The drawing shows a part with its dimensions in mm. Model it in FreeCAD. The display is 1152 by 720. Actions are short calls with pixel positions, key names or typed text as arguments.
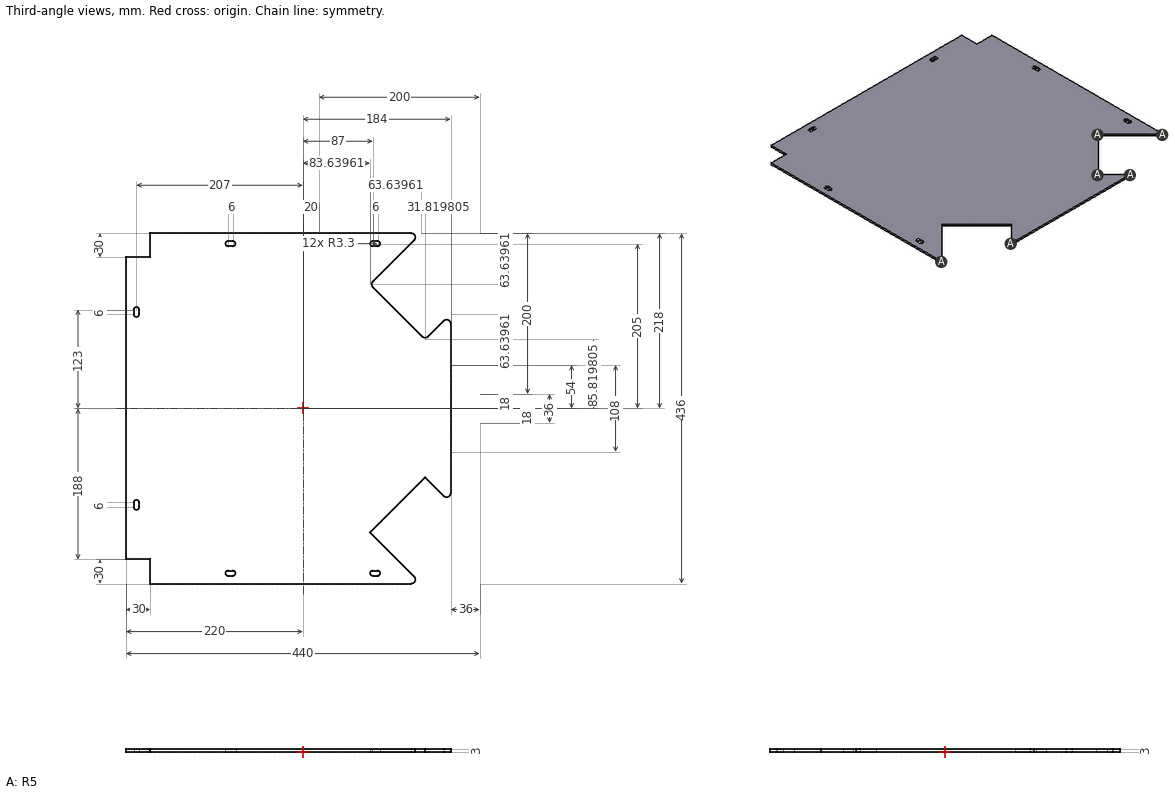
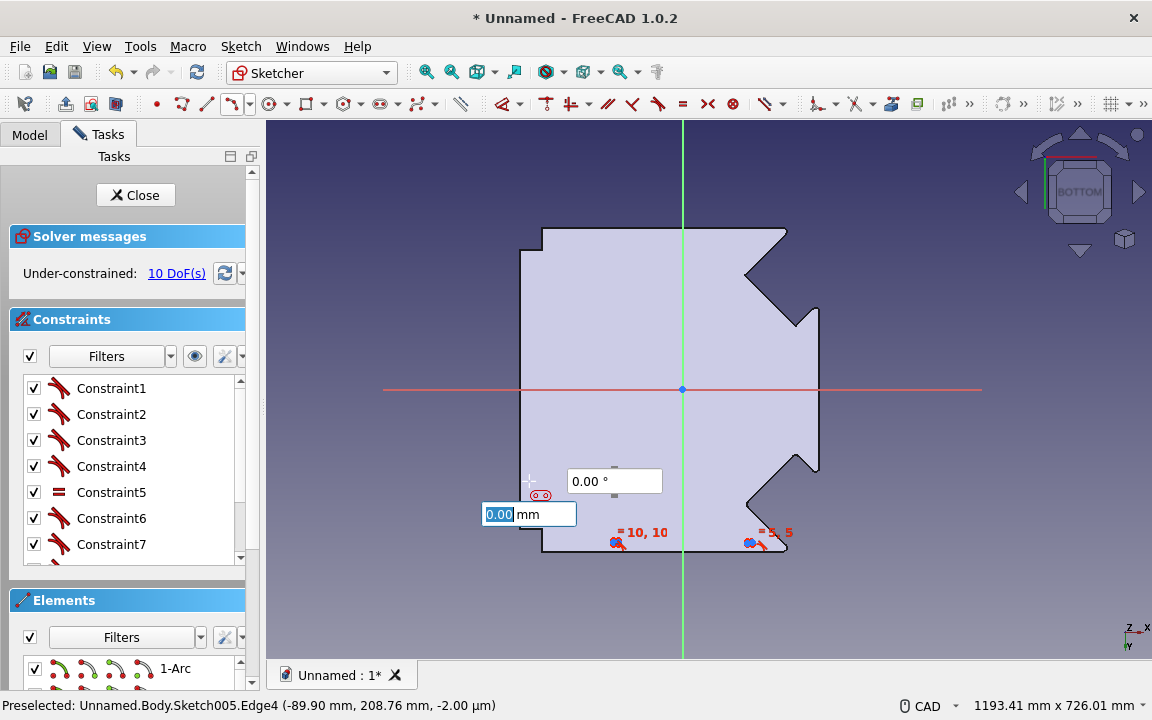
scroll(529, 477, up, 7)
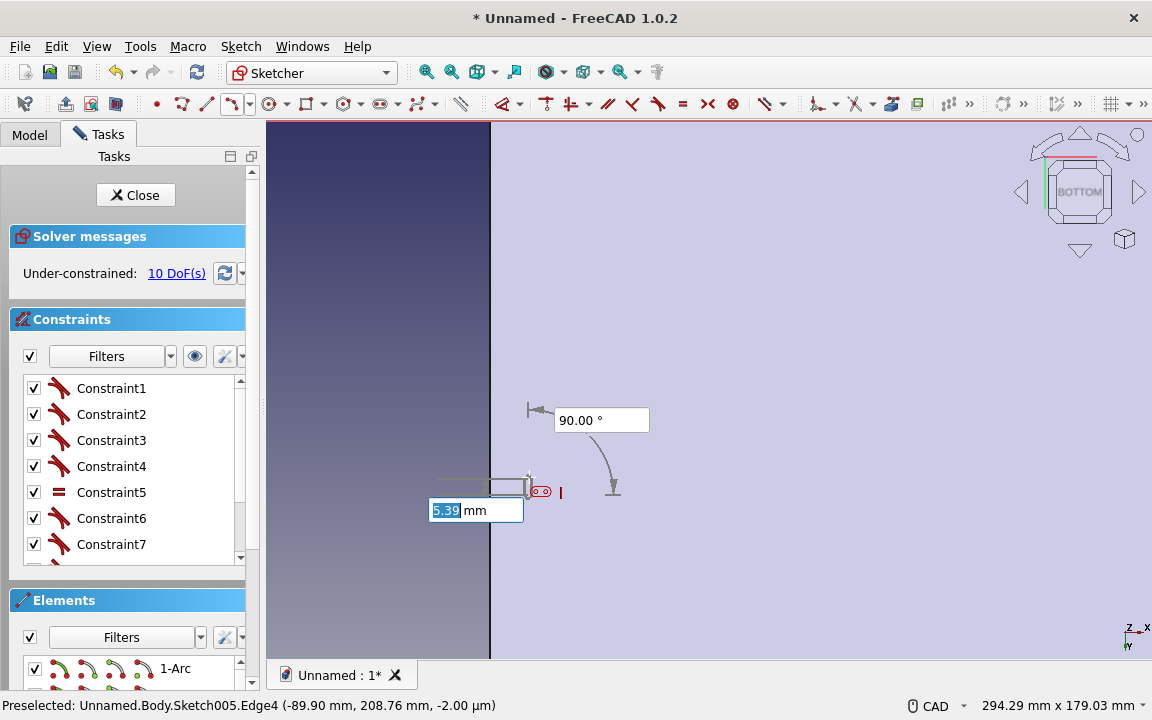
click(528, 474)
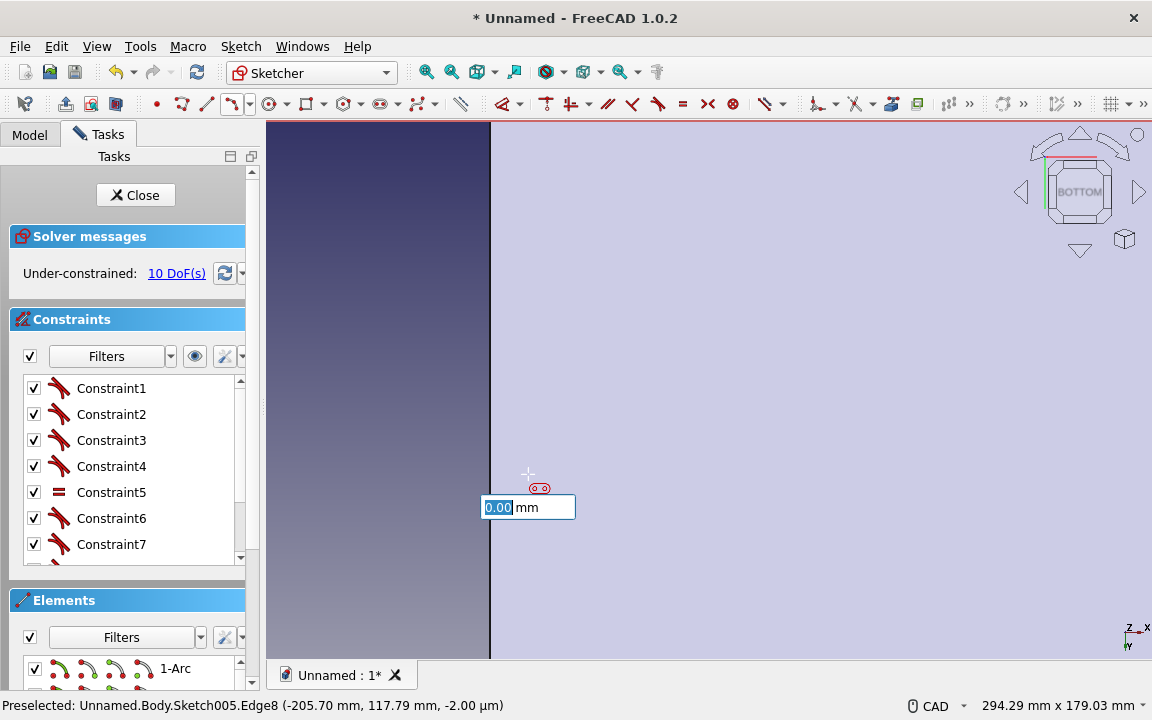
scroll(519, 483, up, 3)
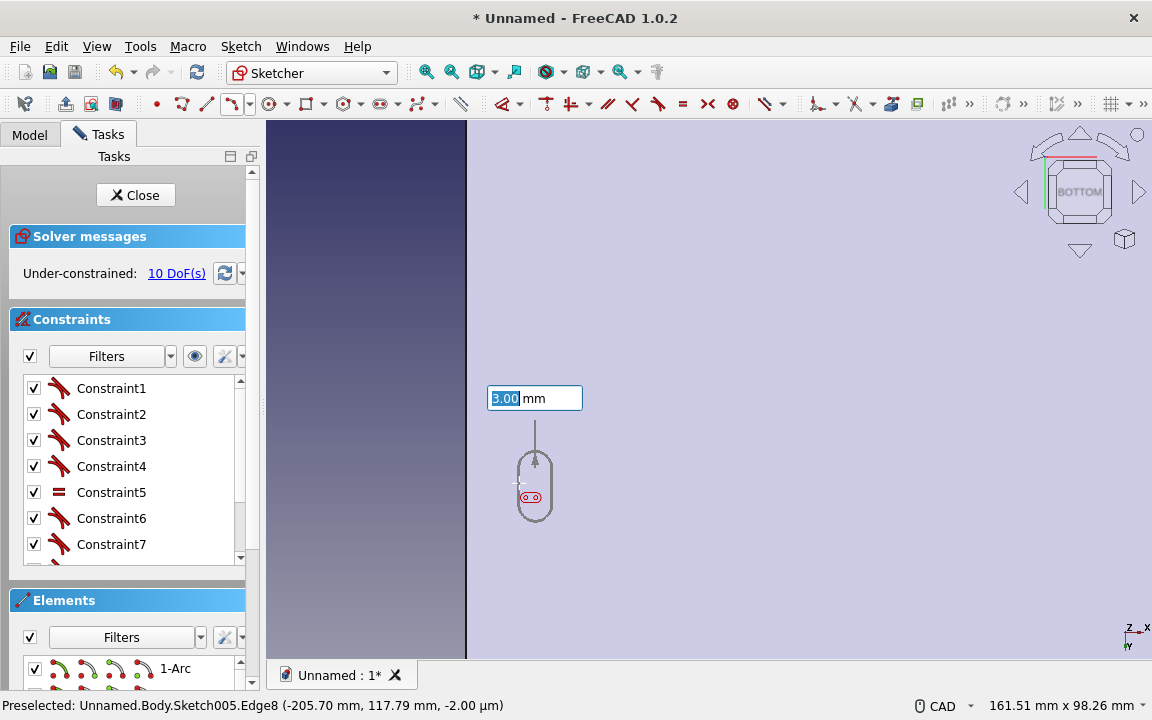
click(519, 482)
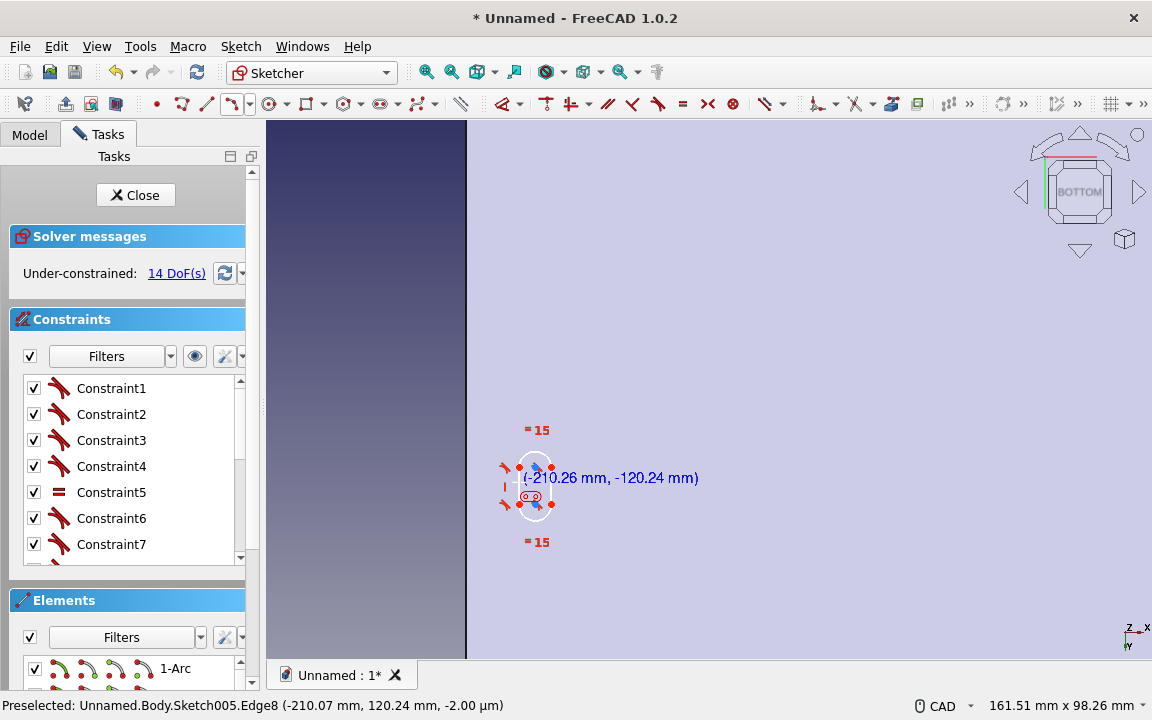
scroll(528, 478, down, 10)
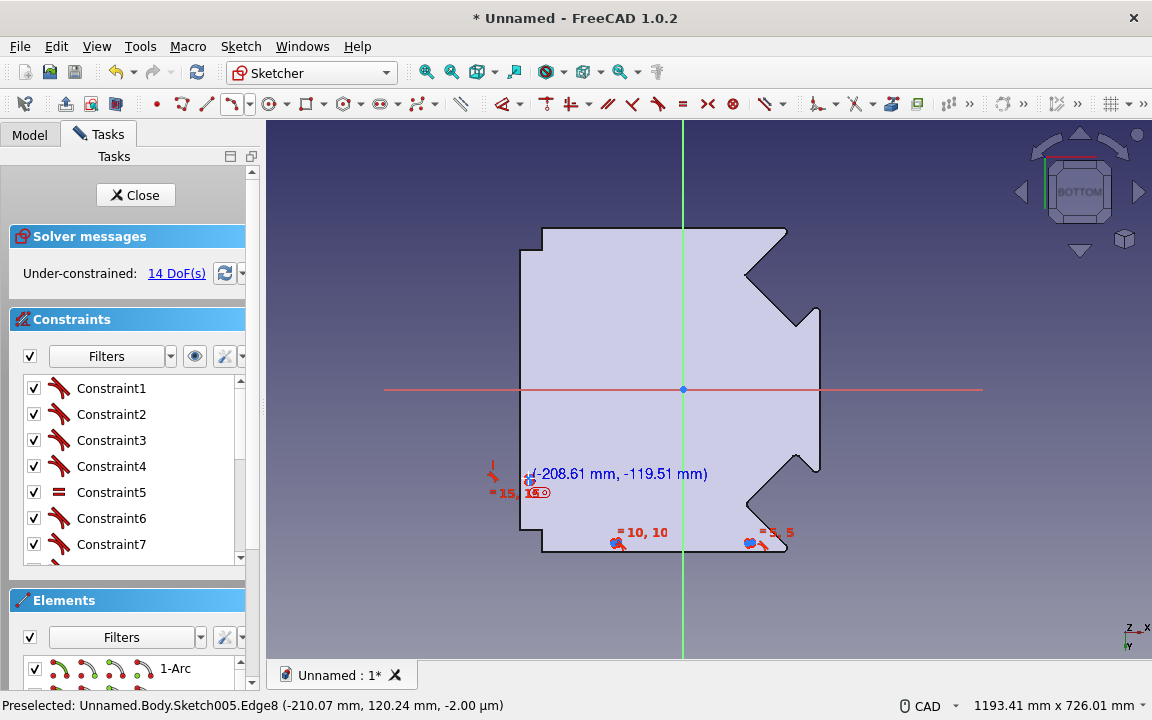
scroll(529, 303, up, 12)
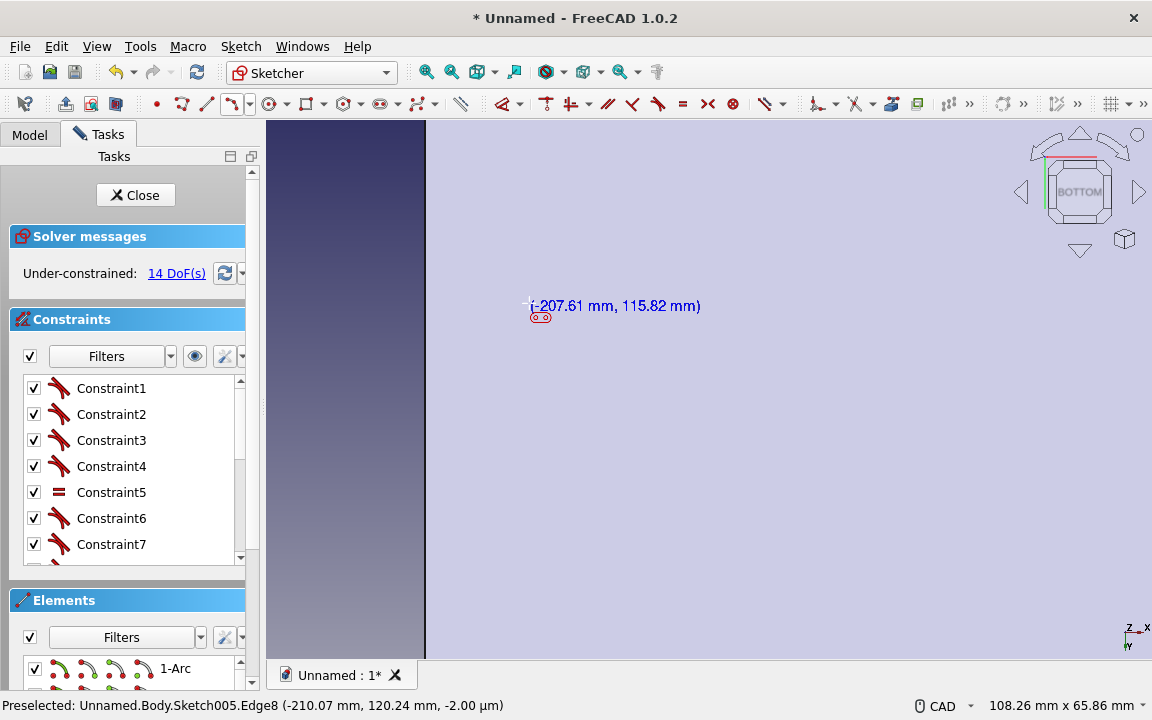
scroll(529, 303, down, 12)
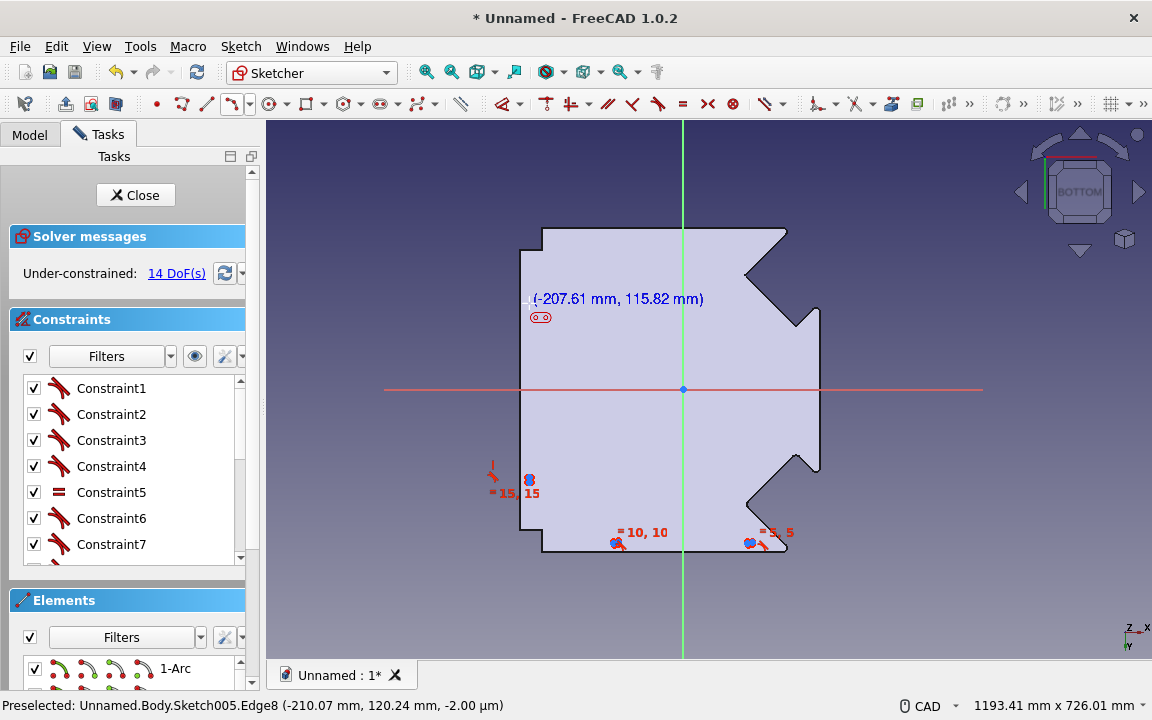
click(529, 303)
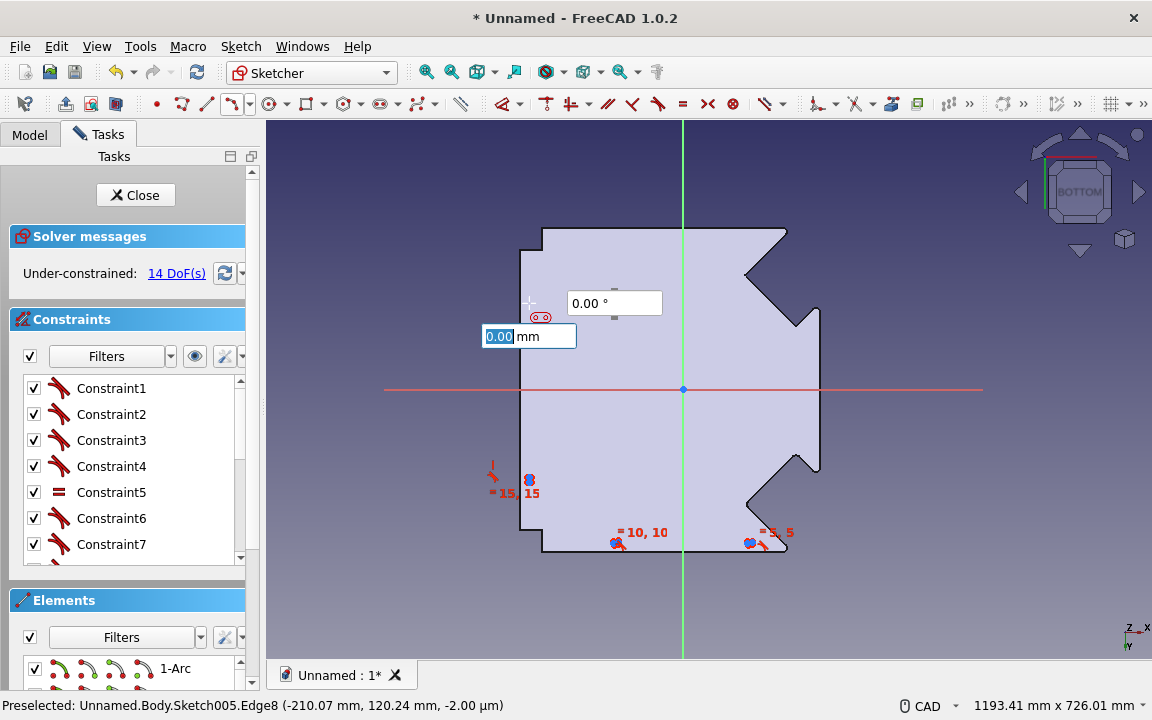
scroll(529, 299, up, 7)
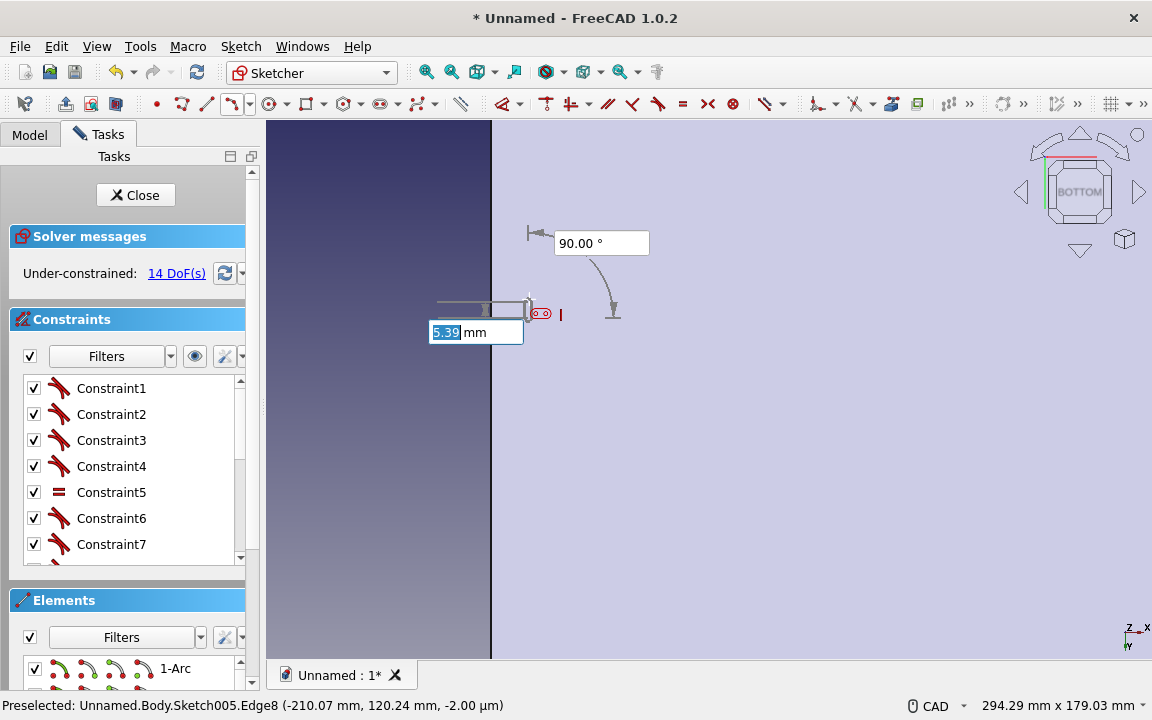
click(528, 297)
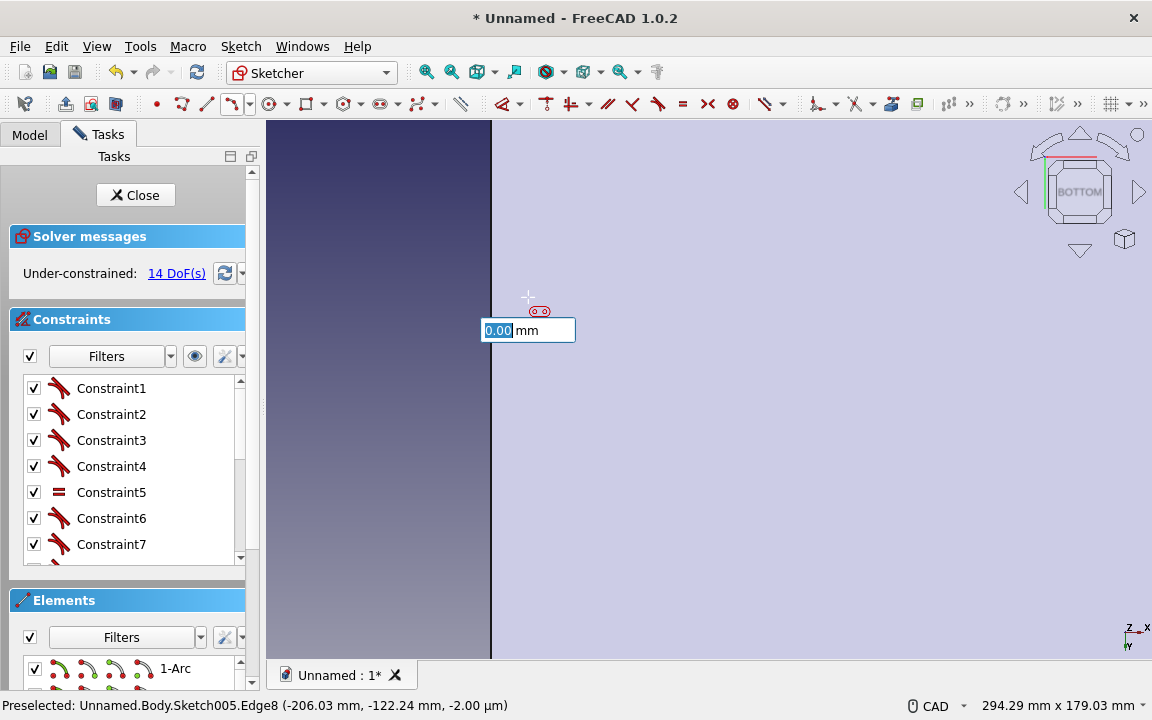
scroll(520, 306, up, 3)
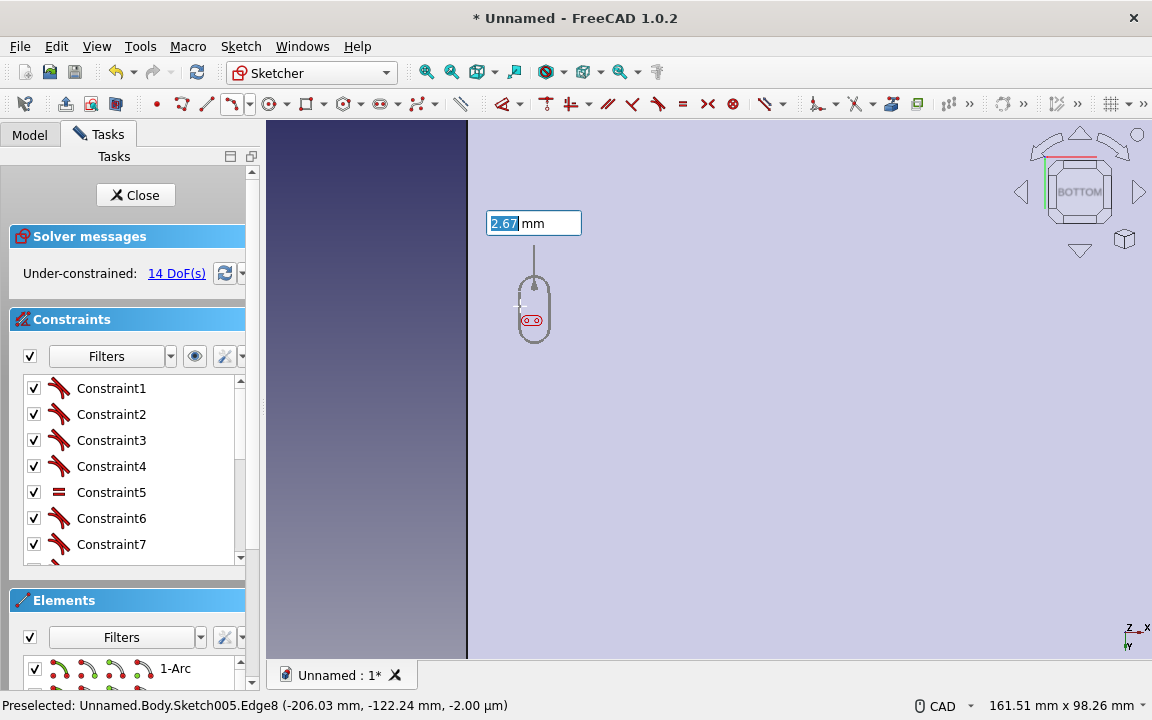
click(520, 305)